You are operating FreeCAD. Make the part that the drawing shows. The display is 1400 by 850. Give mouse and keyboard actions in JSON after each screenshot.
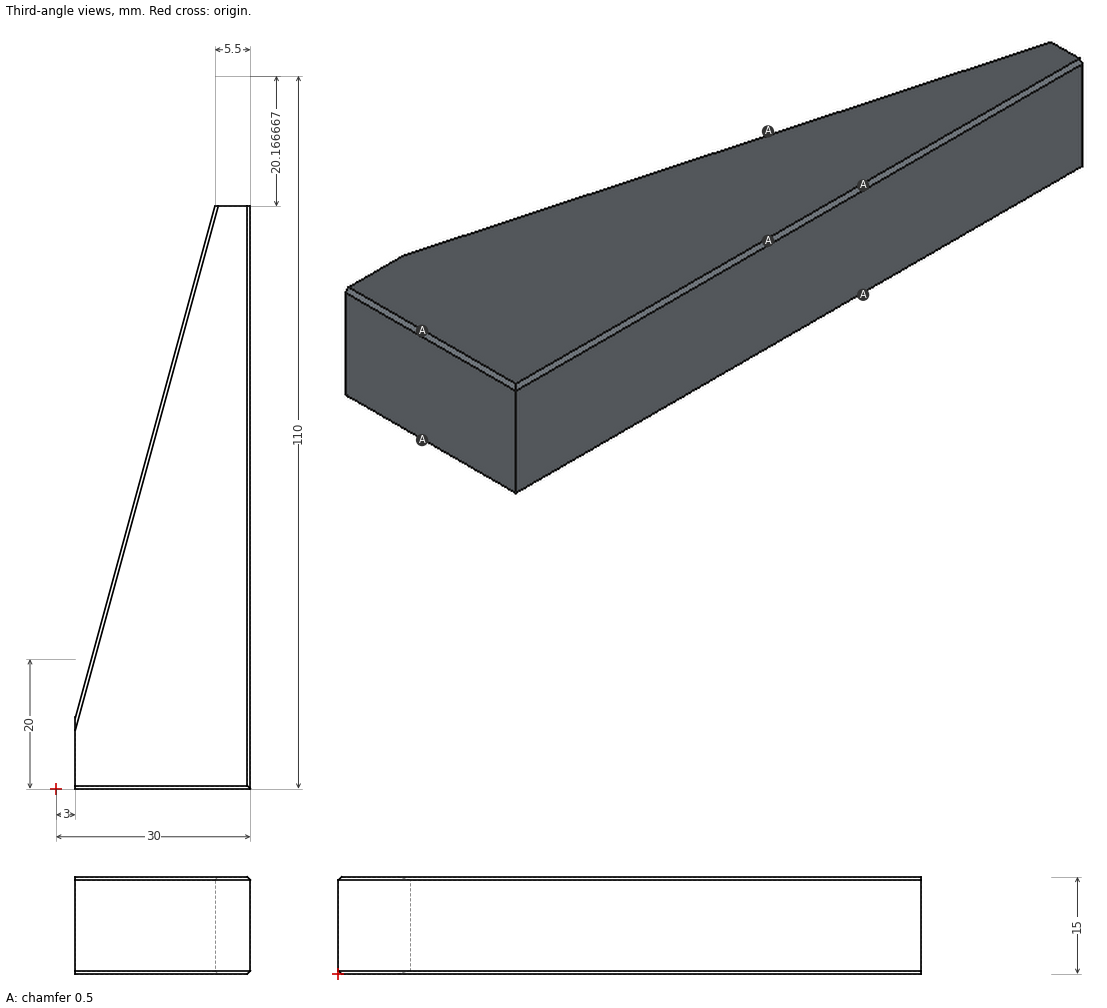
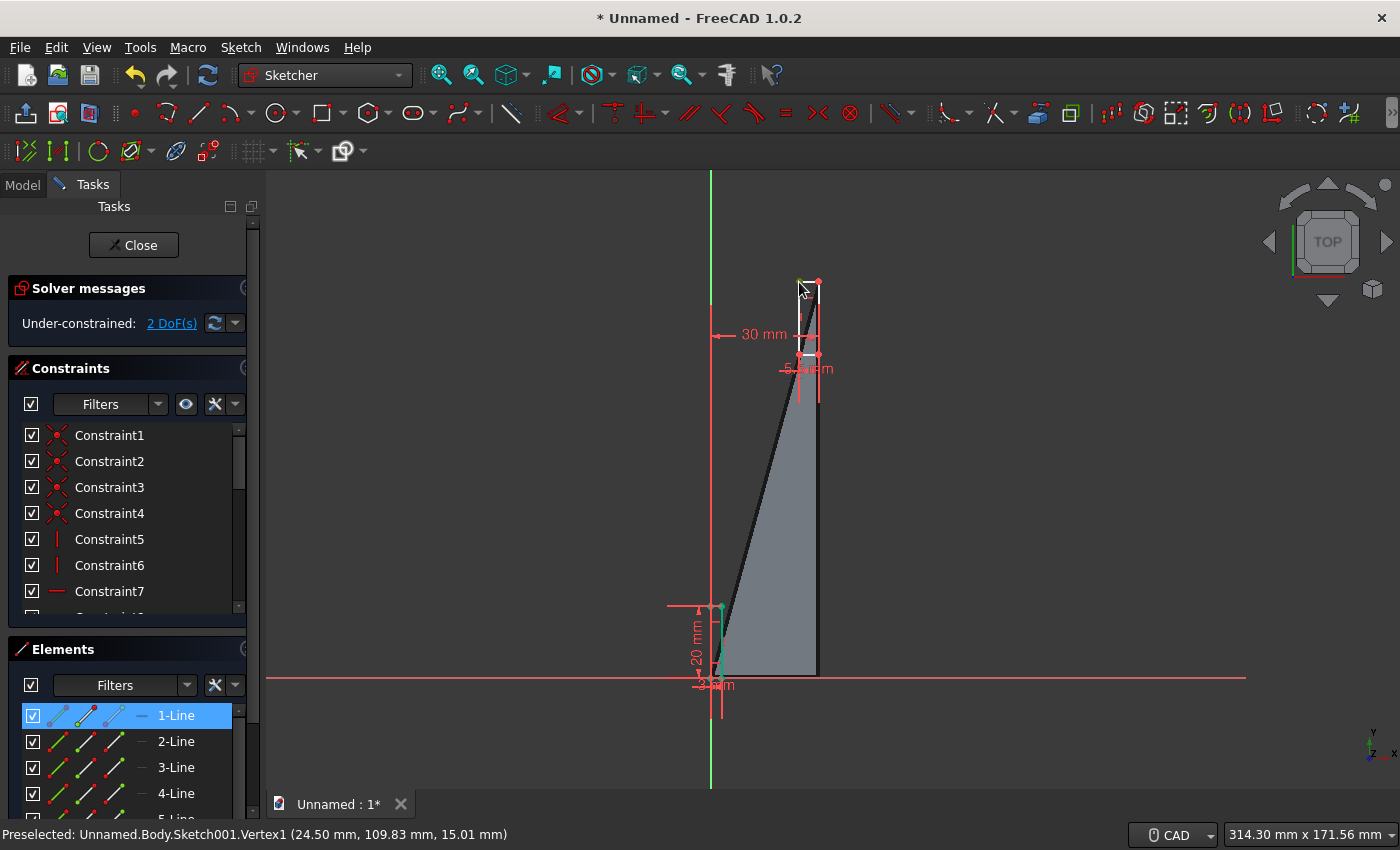
{"action": "key", "text": "i"}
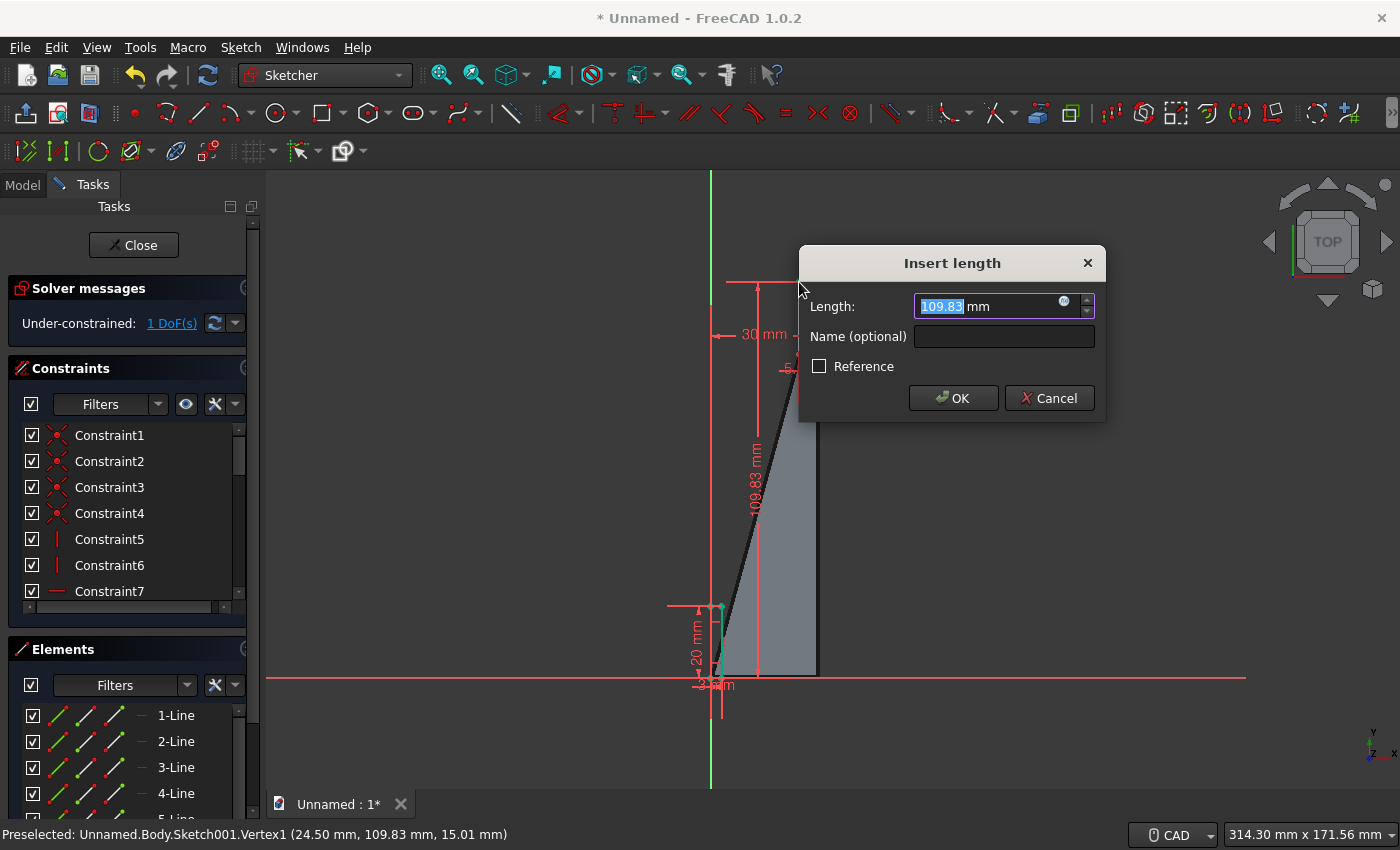
{"action": "type", "text": "110"}
{"action": "key", "text": "Return"}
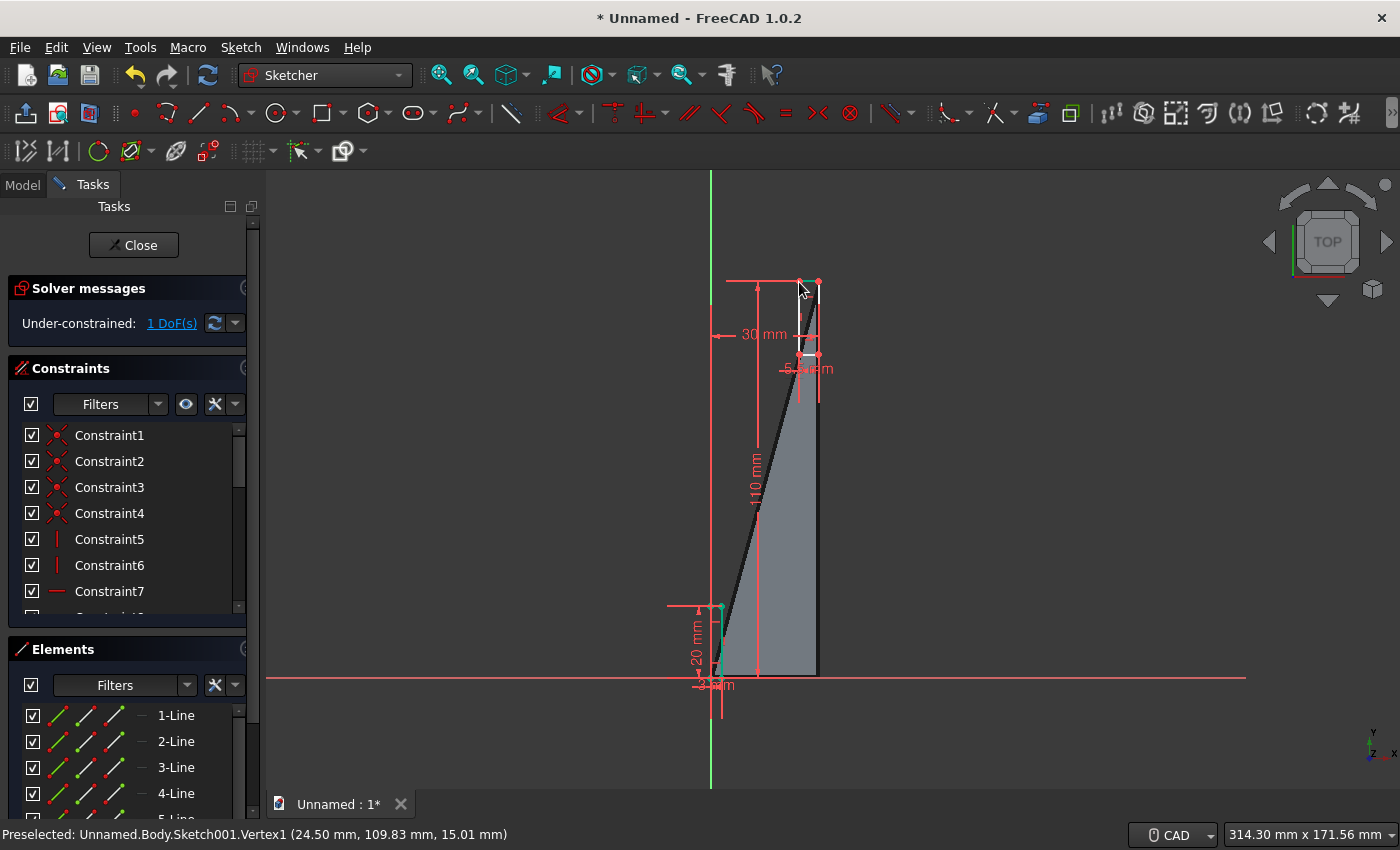
{"action": "left_click", "coordinate": [799, 303]}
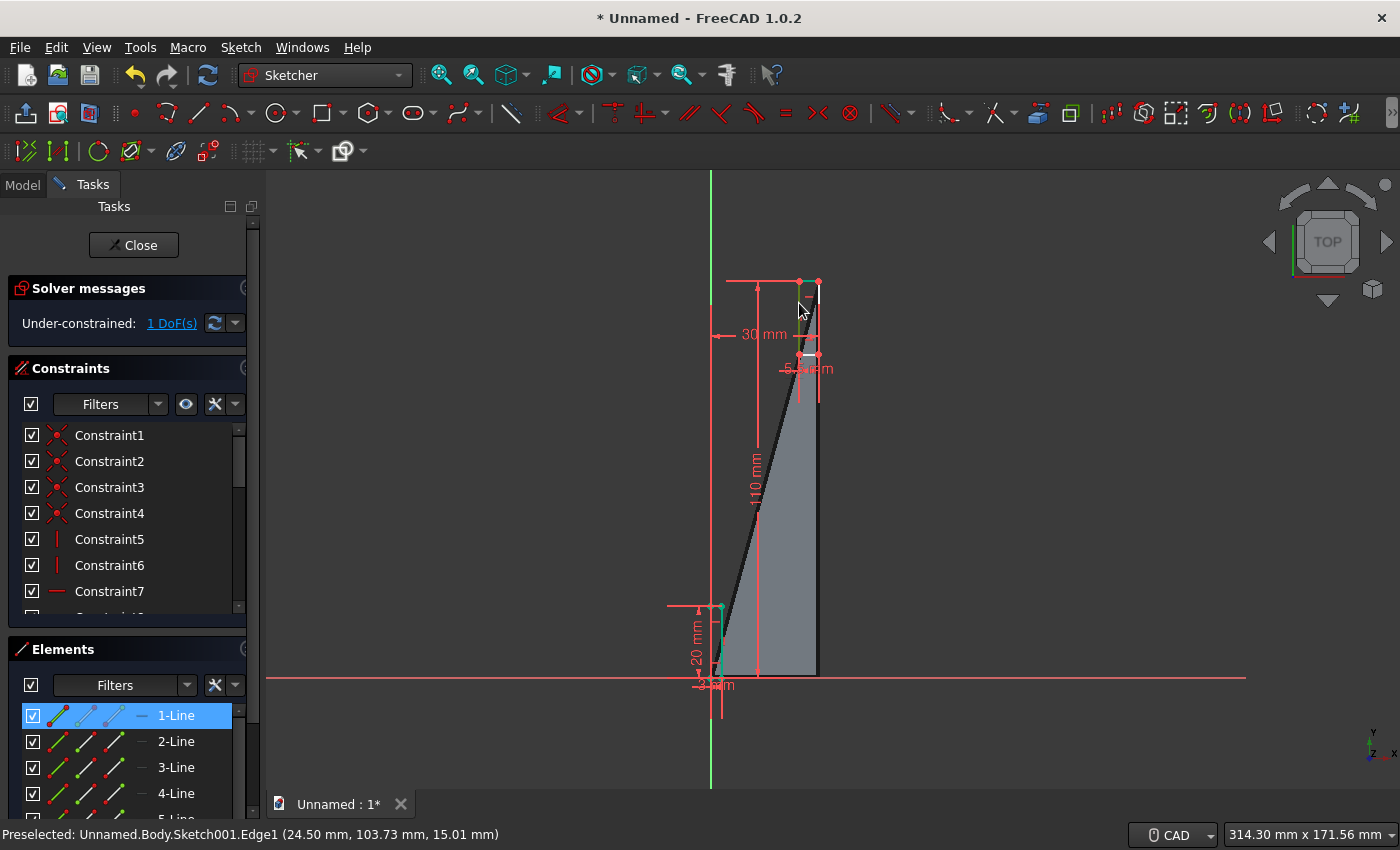
{"action": "key", "text": "i"}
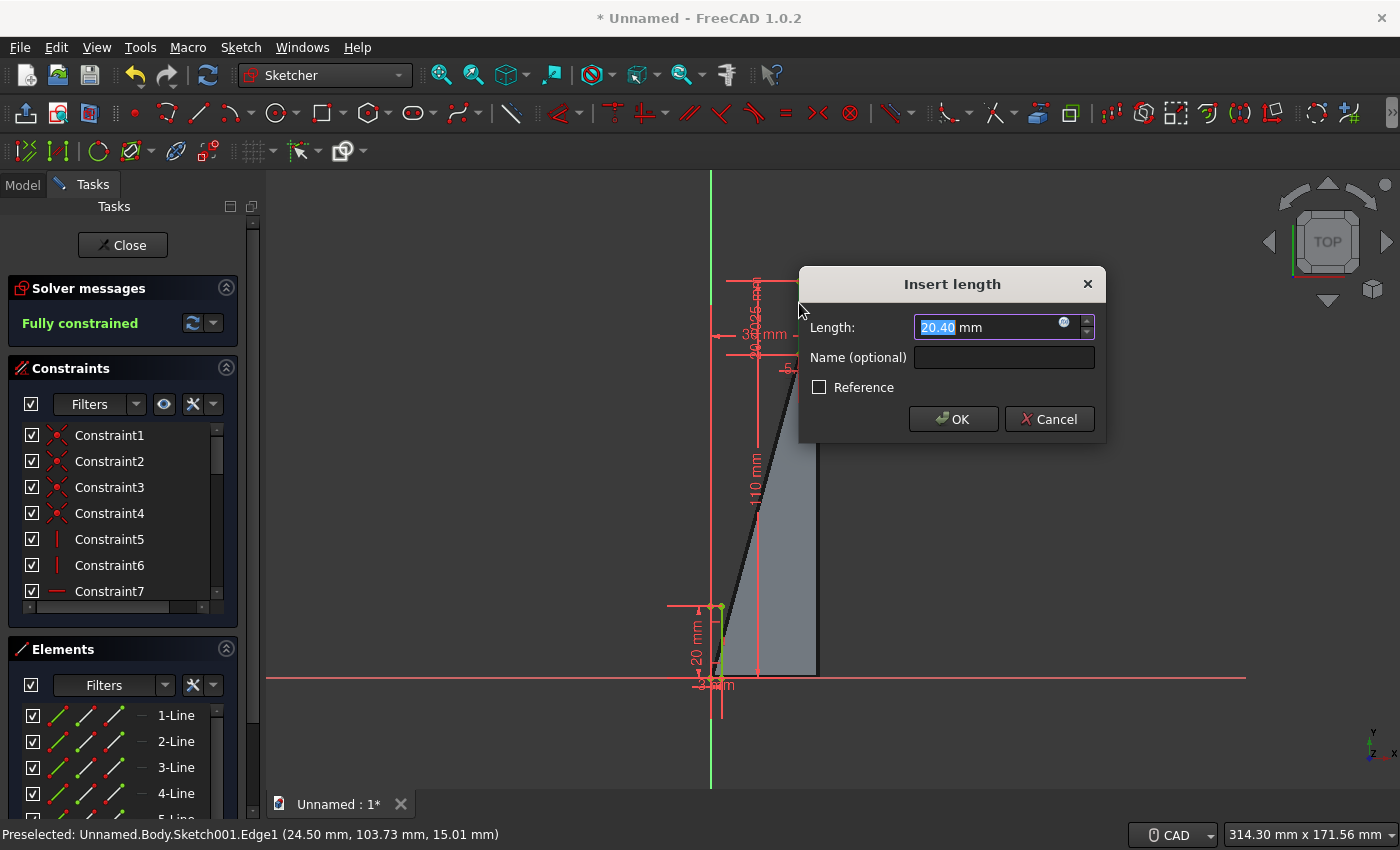
{"action": "type", "text": "20.166667"}
{"action": "key", "text": "Return"}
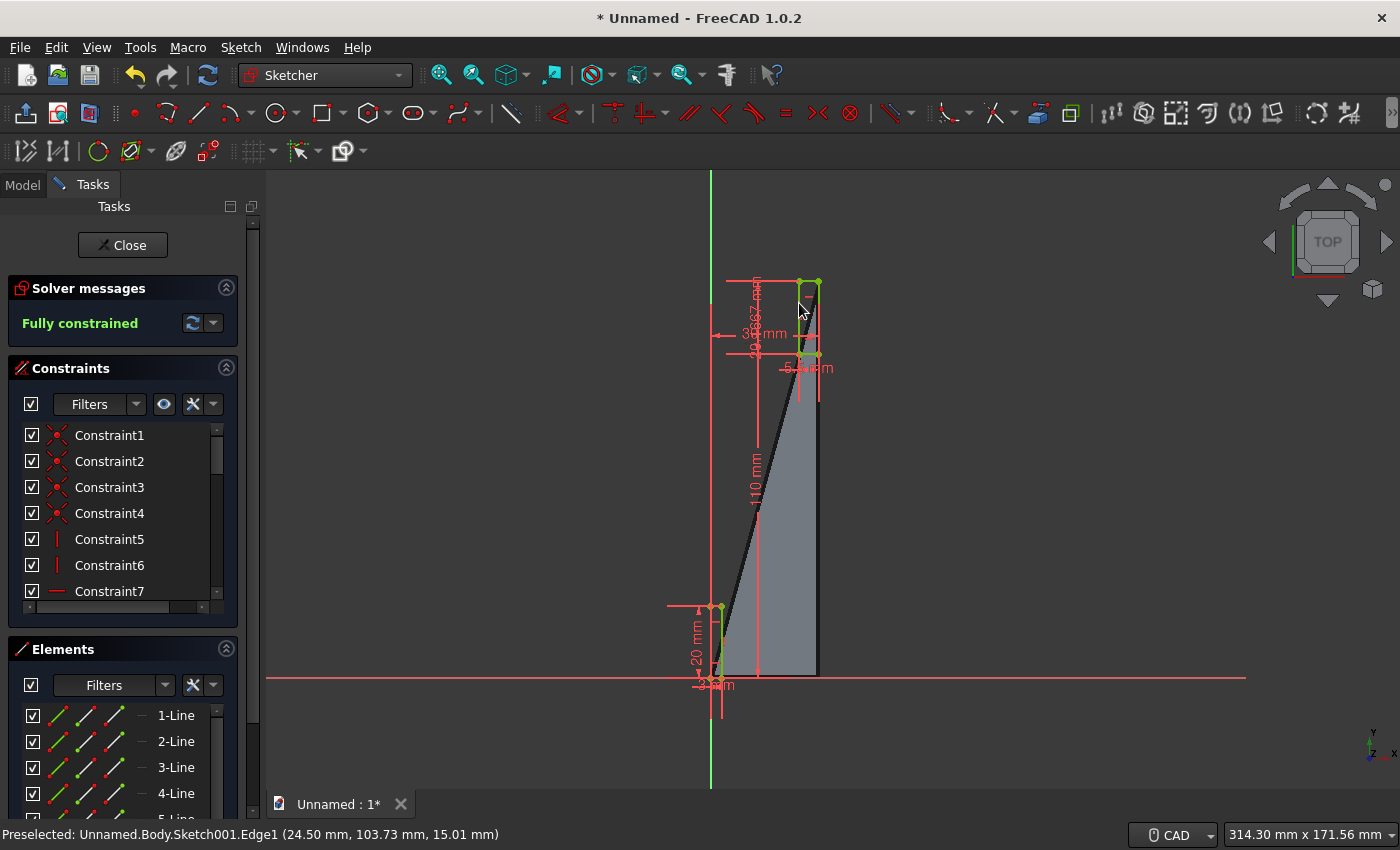
{"action": "left_click", "coordinate": [123, 245]}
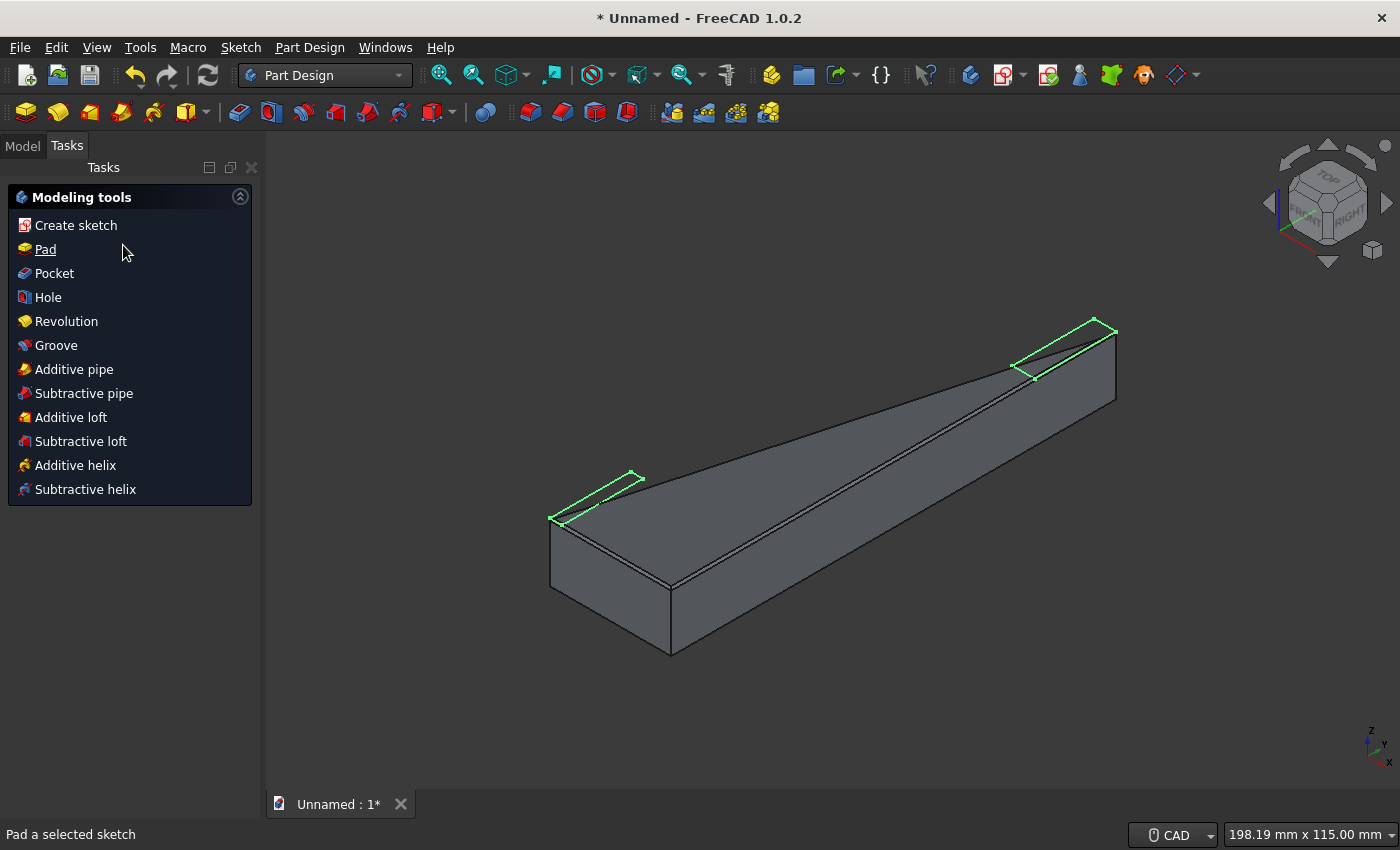
{"action": "left_click", "coordinate": [240, 112]}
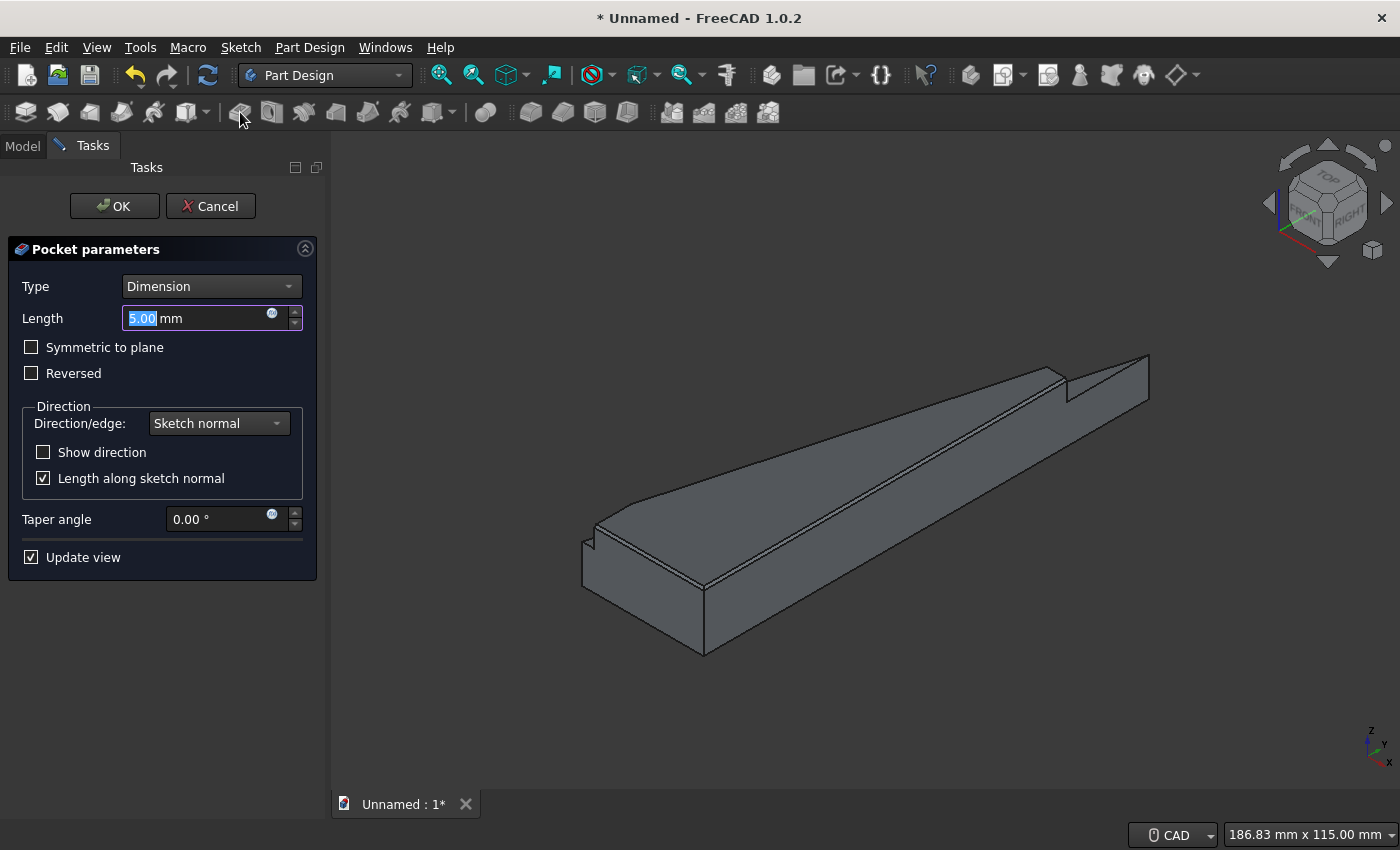
{"action": "left_click", "coordinate": [212, 286]}